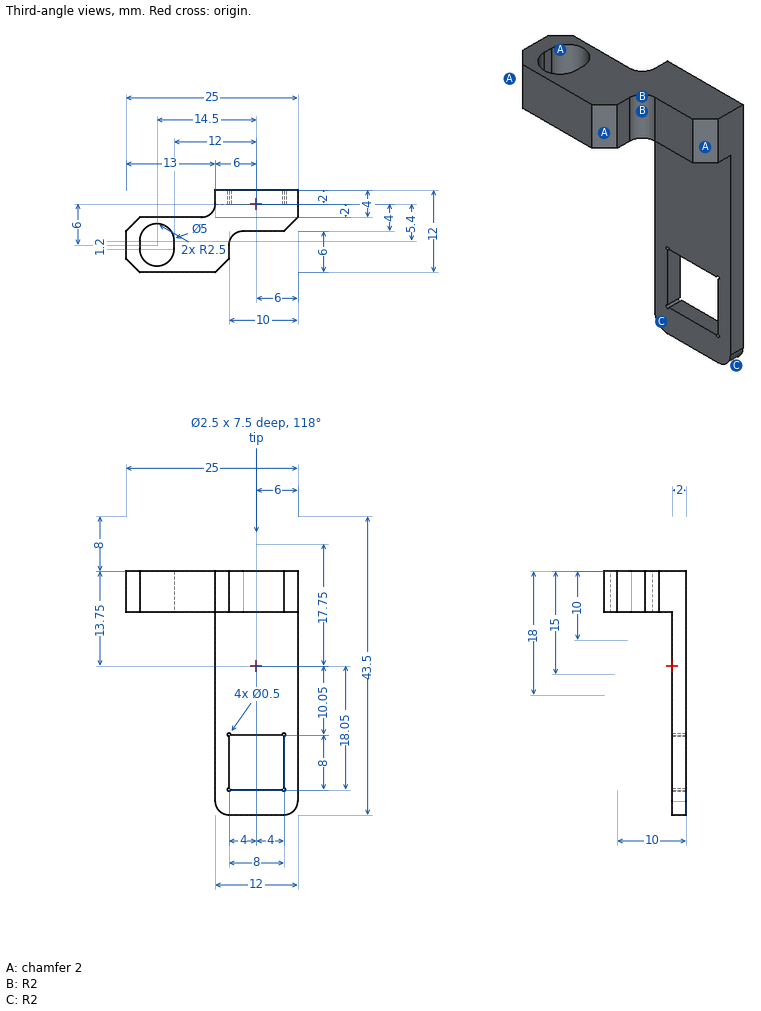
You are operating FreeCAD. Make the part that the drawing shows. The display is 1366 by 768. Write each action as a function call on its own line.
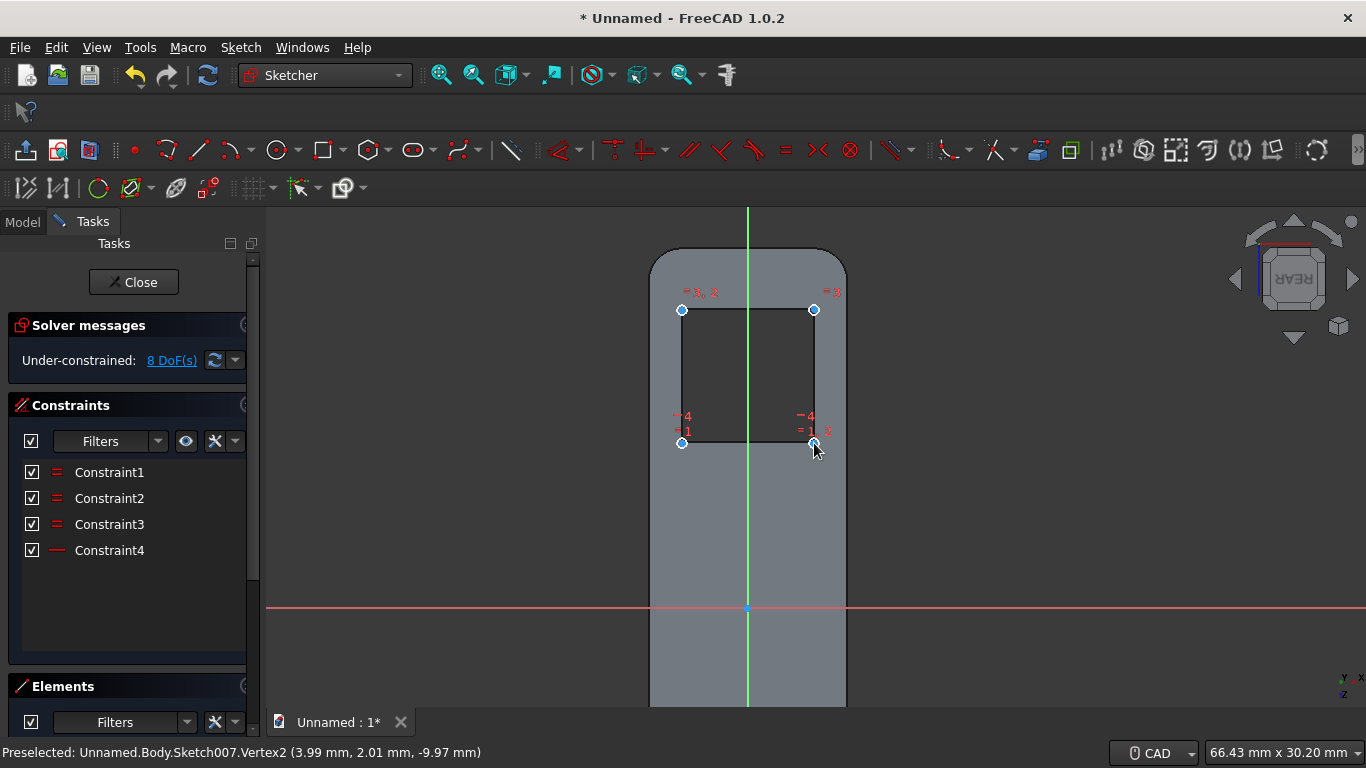
click(682, 443)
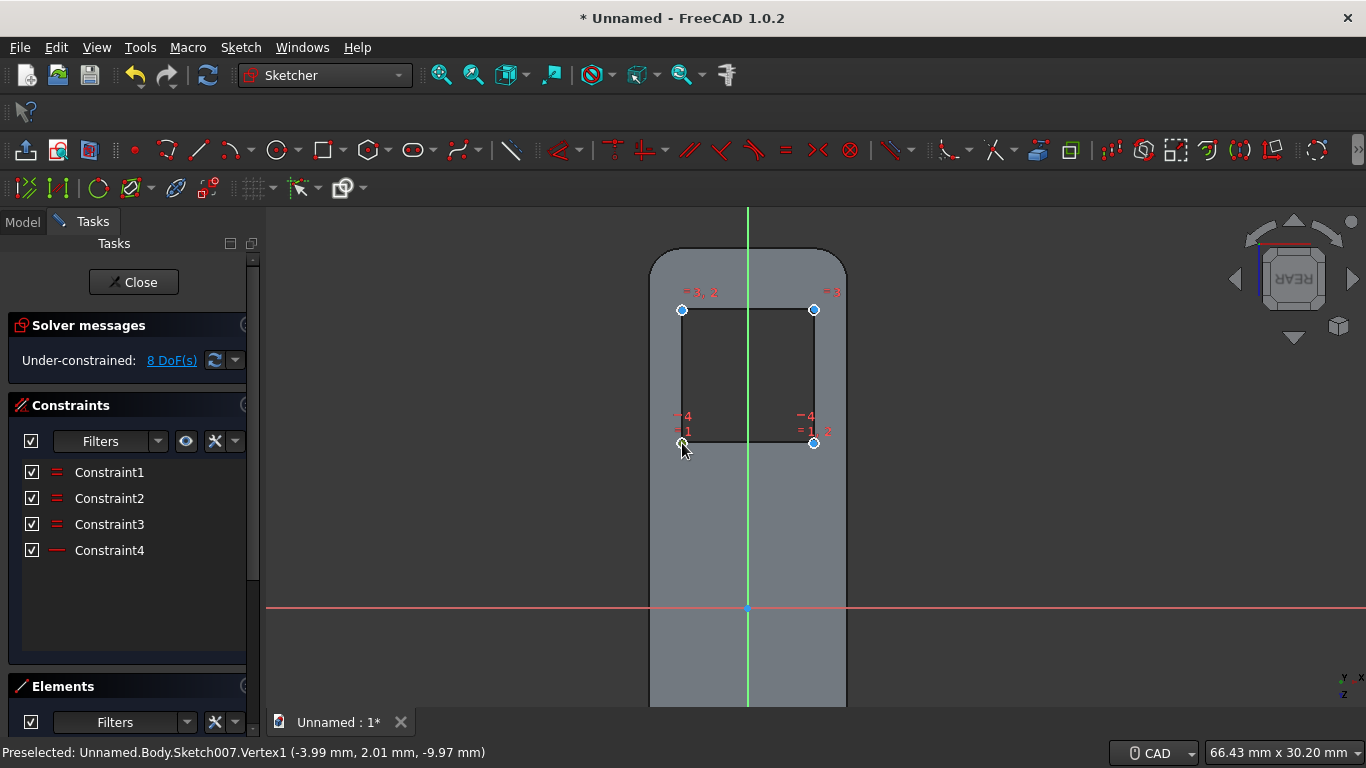
click(682, 310)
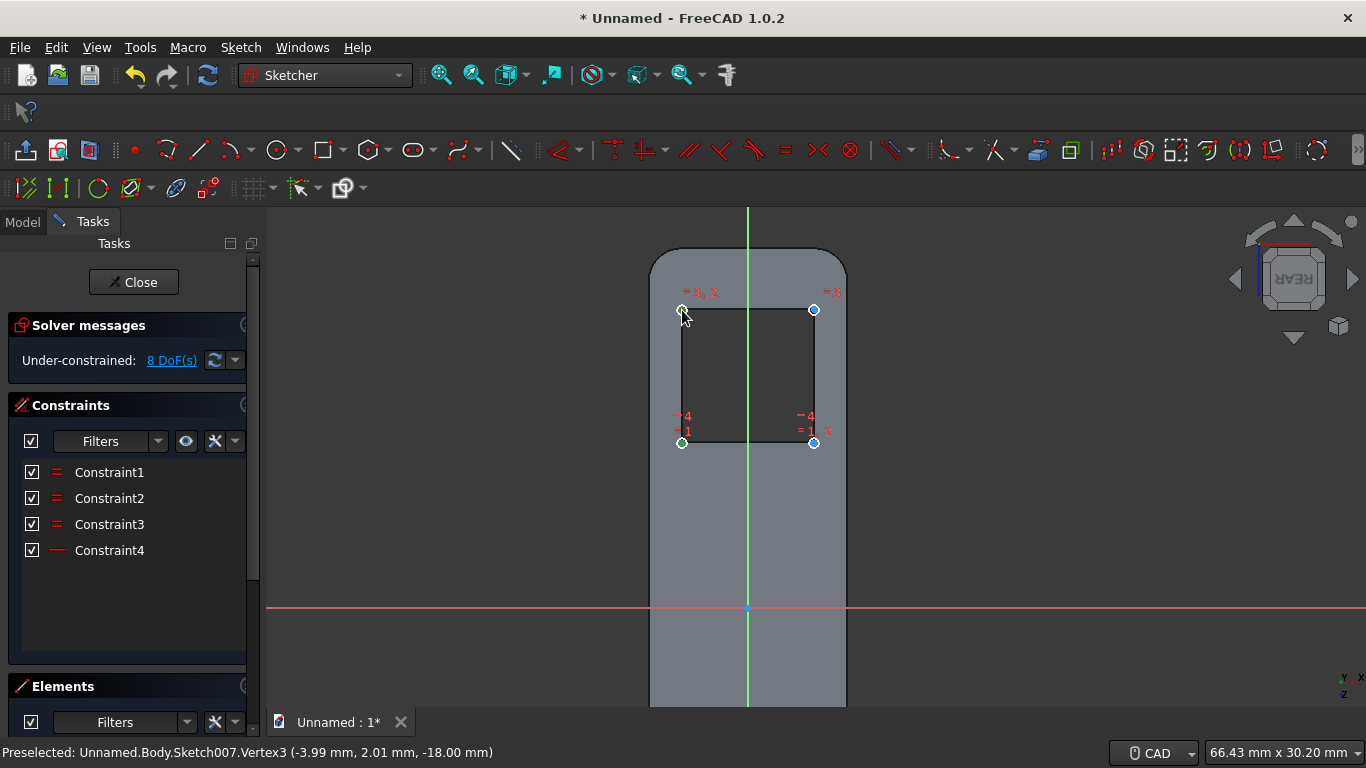
key(v)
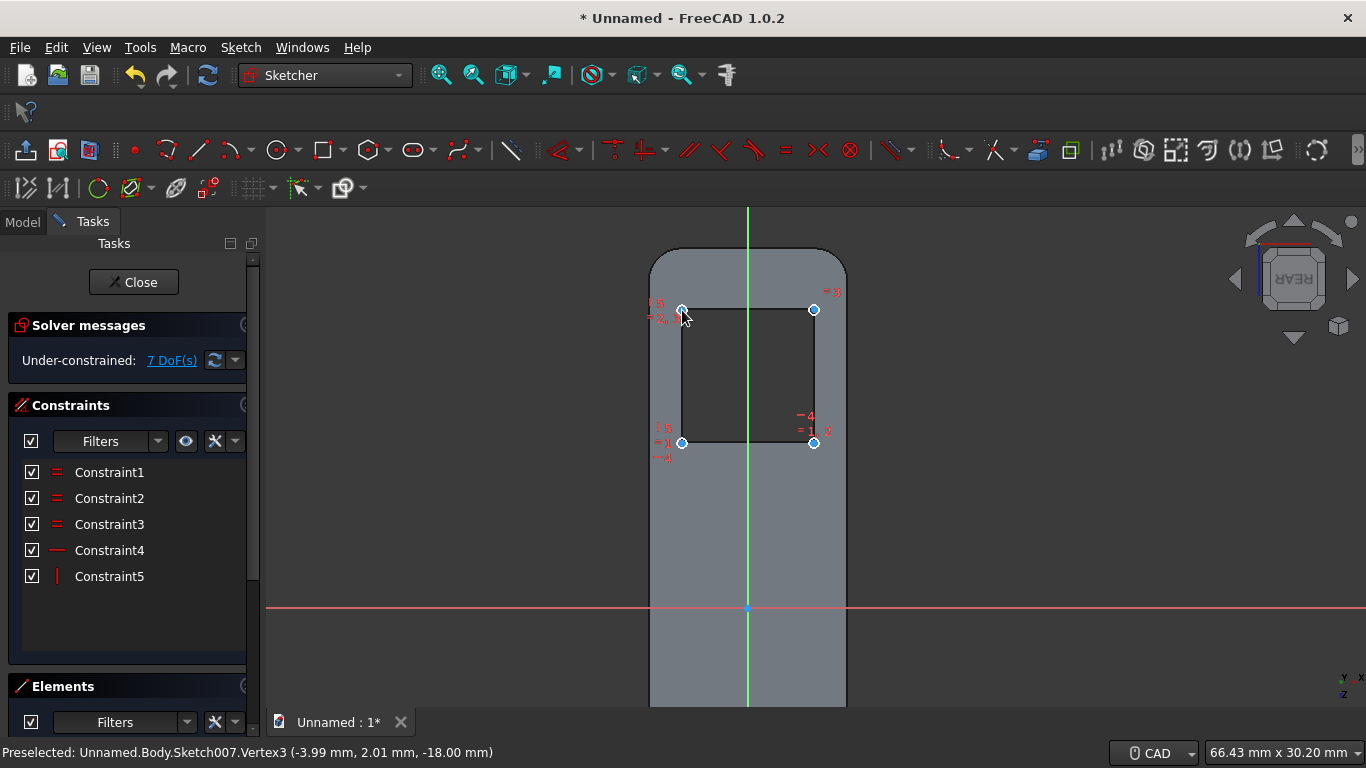
click(814, 443)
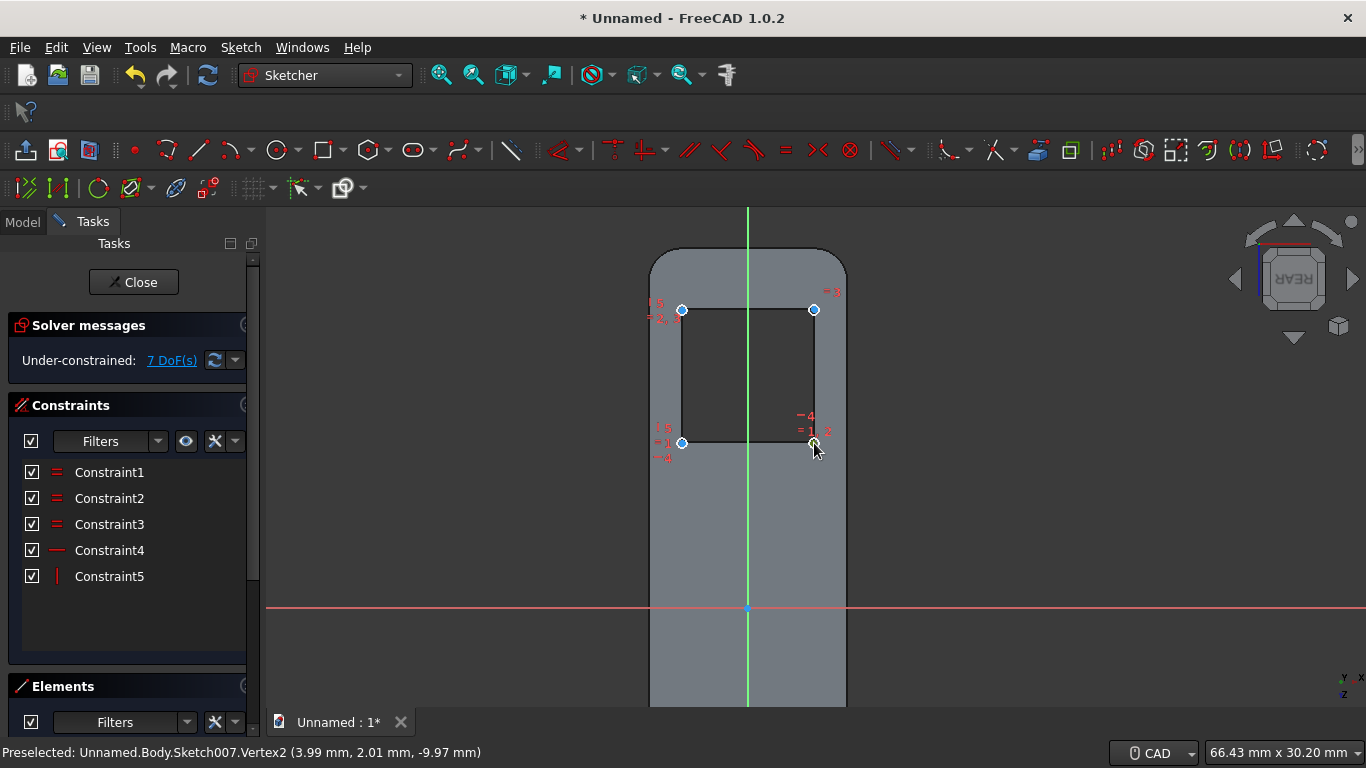
click(814, 310)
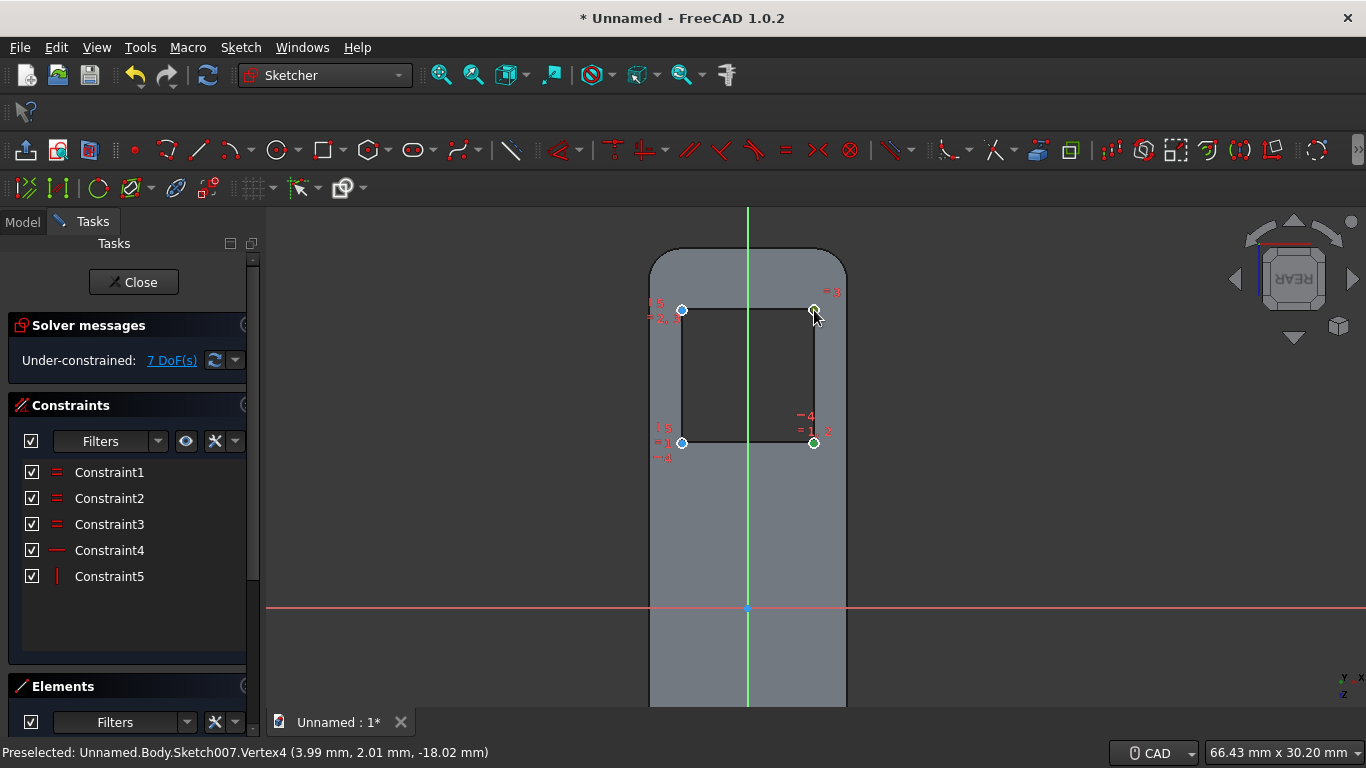
click(668, 150)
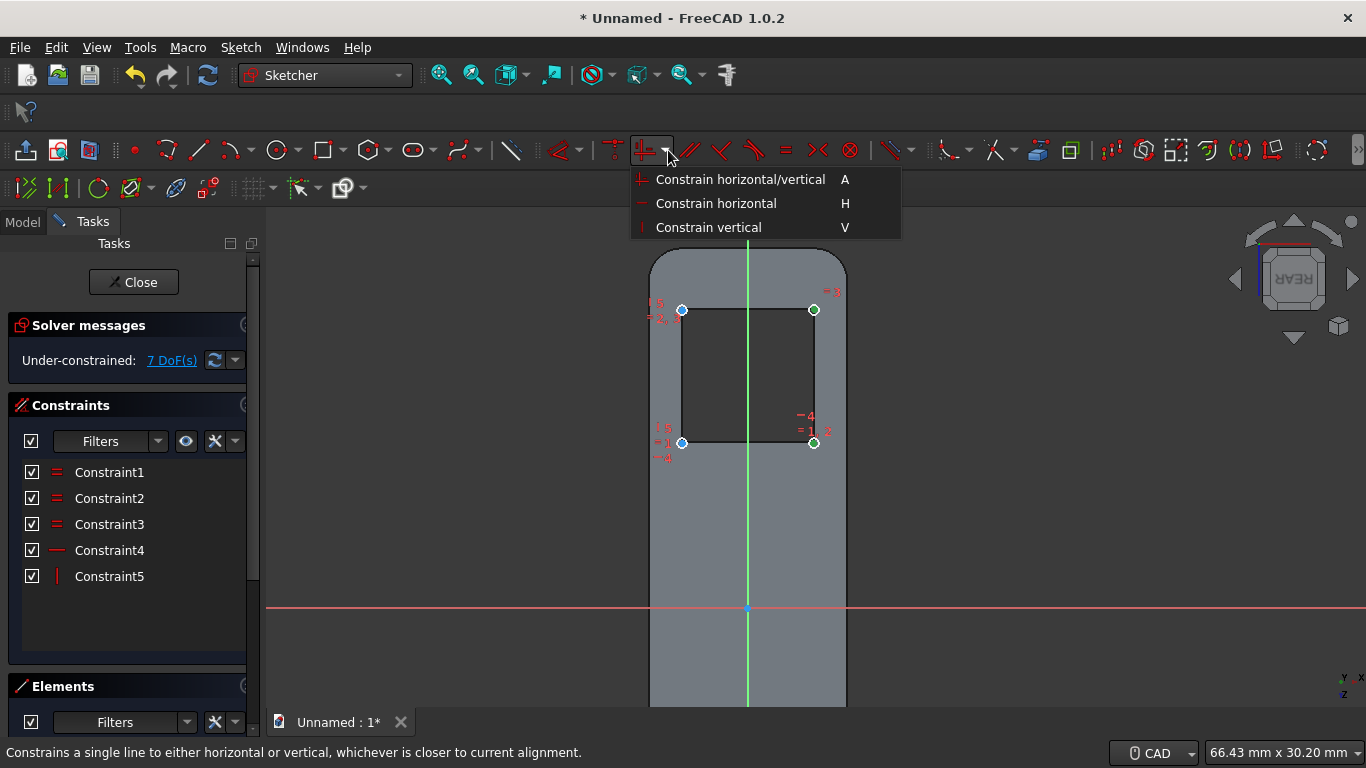
click(766, 227)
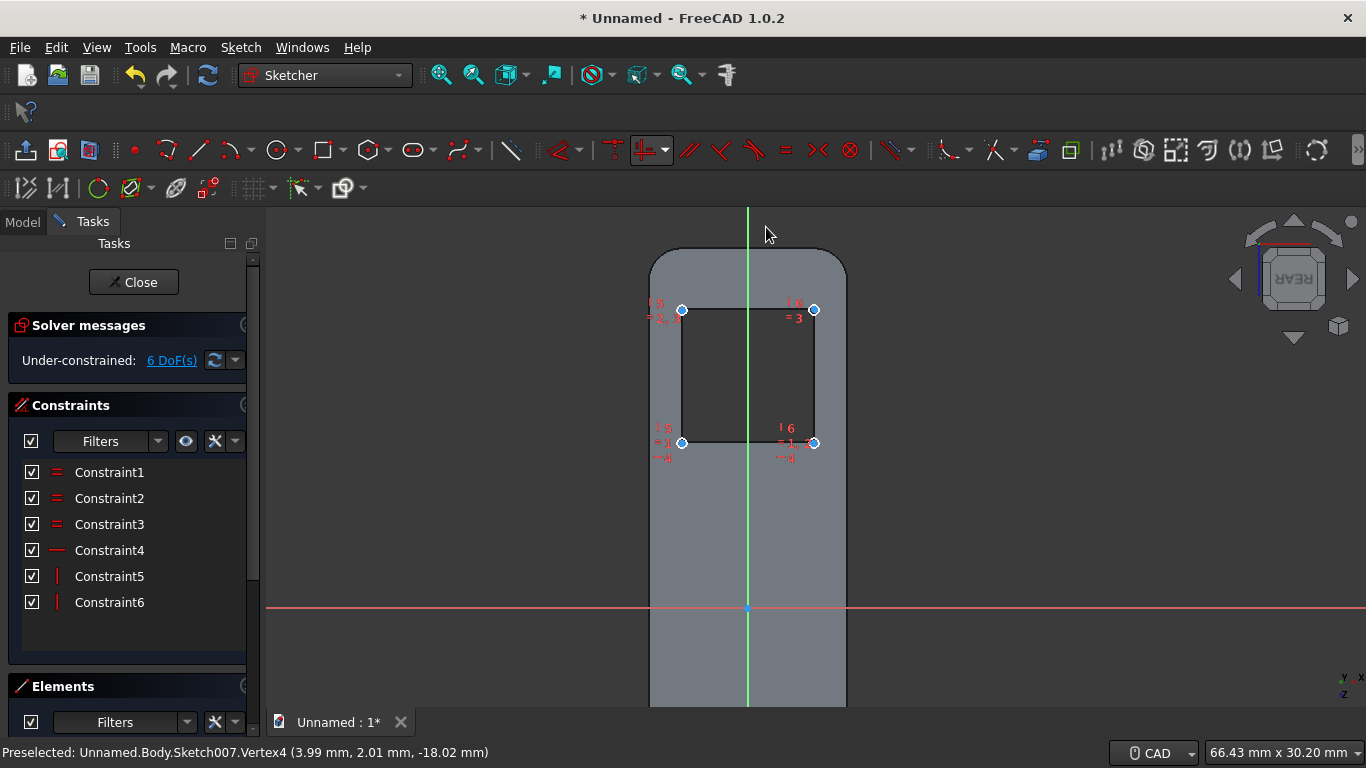
click(682, 310)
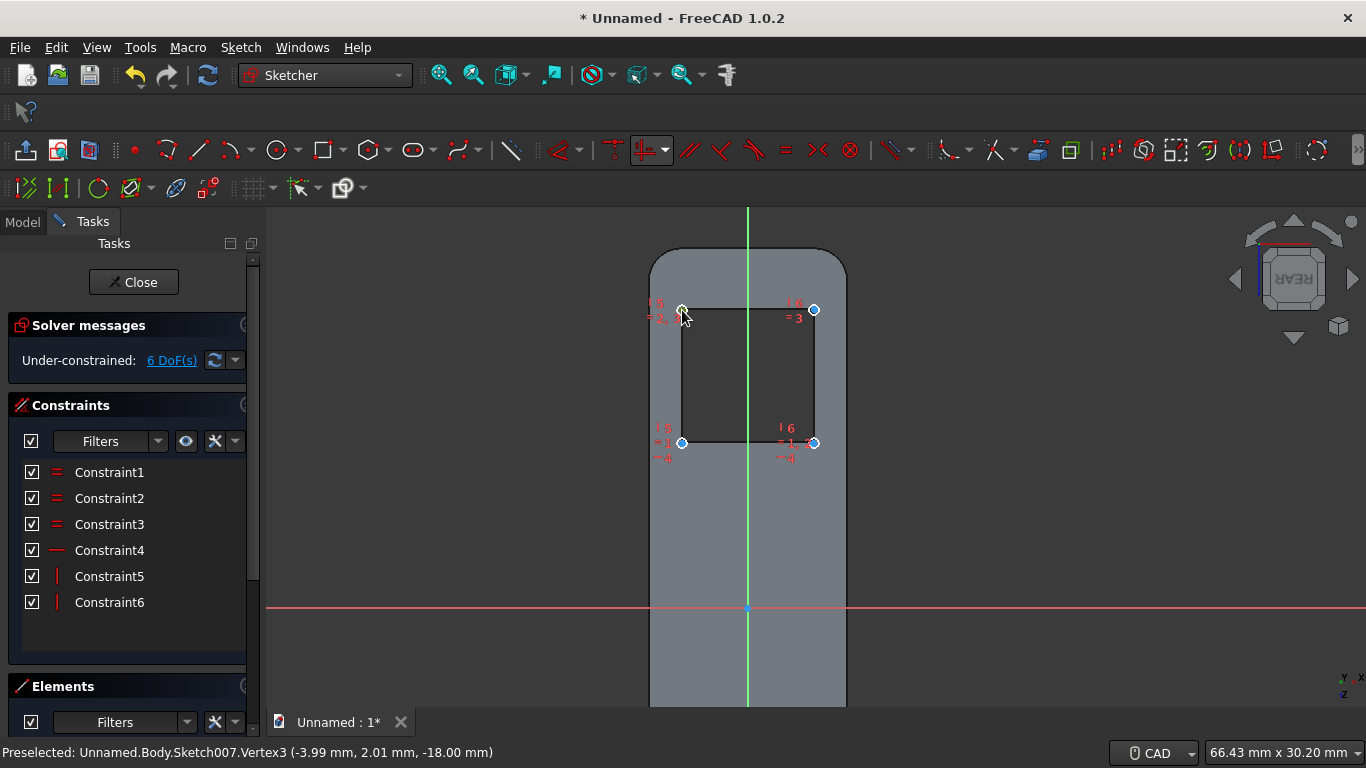
click(814, 310)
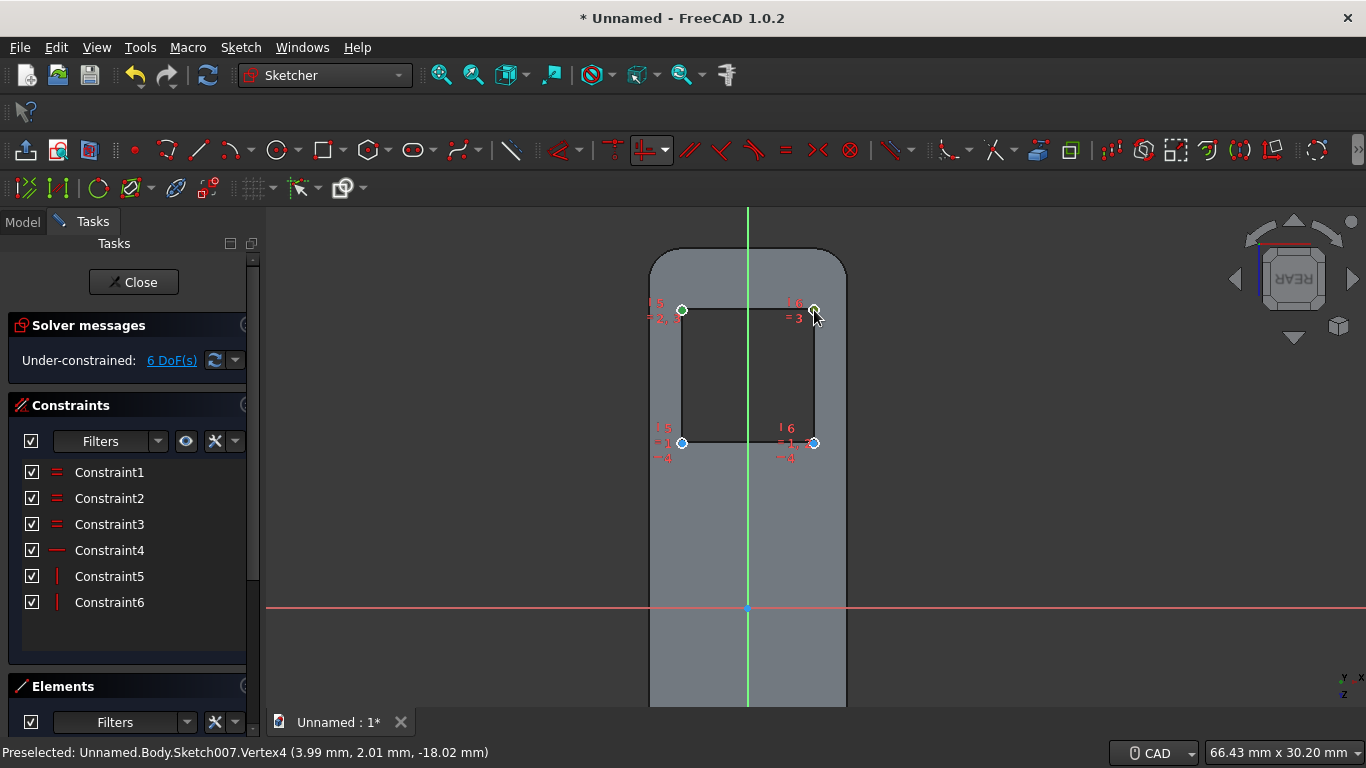
click(668, 150)